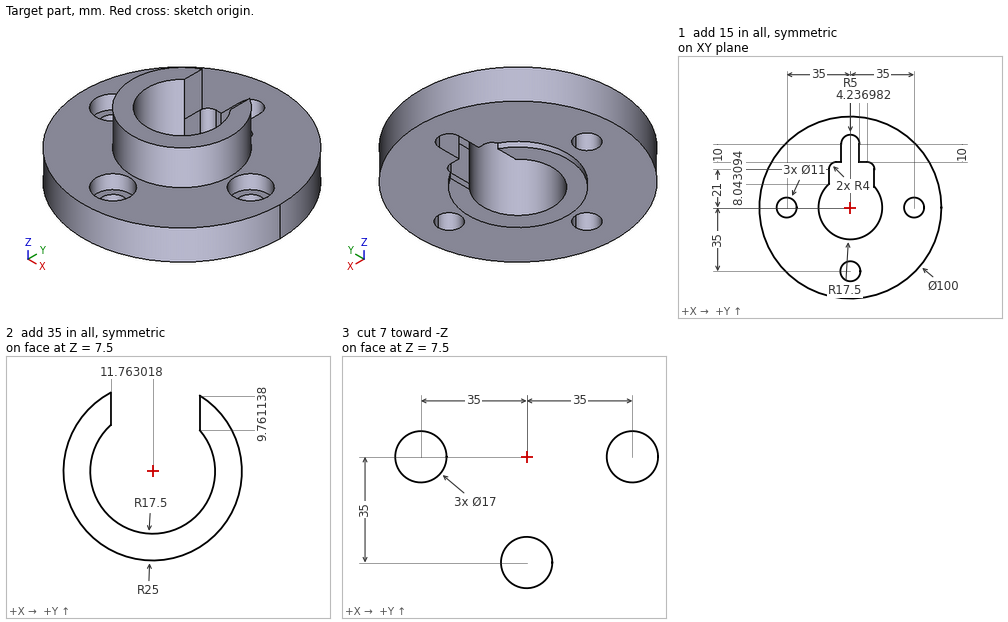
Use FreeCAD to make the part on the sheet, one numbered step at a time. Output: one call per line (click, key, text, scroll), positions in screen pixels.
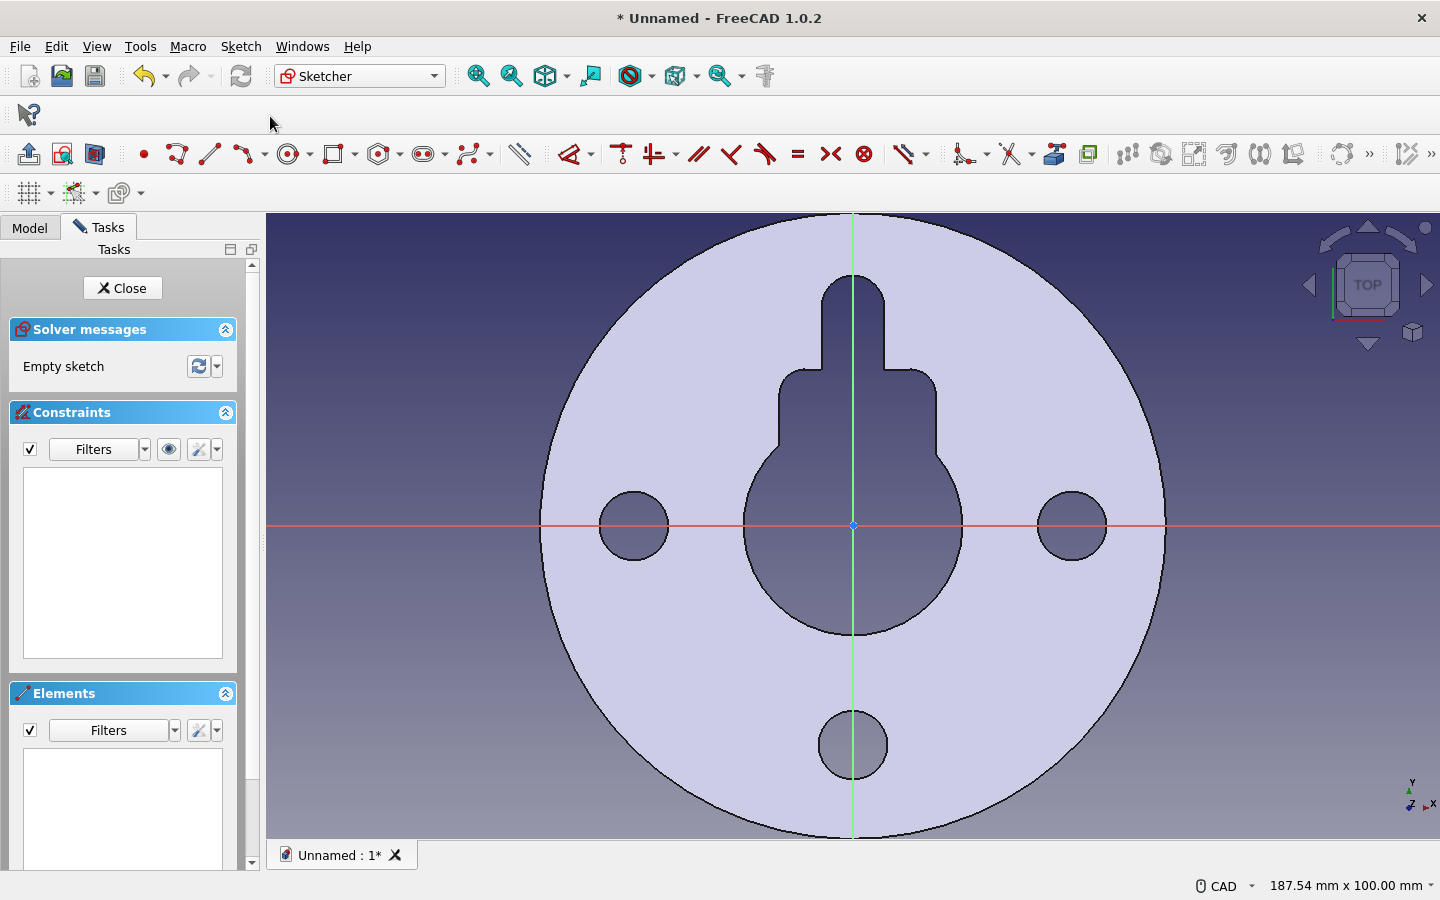
scroll(1006, 554, up, 2)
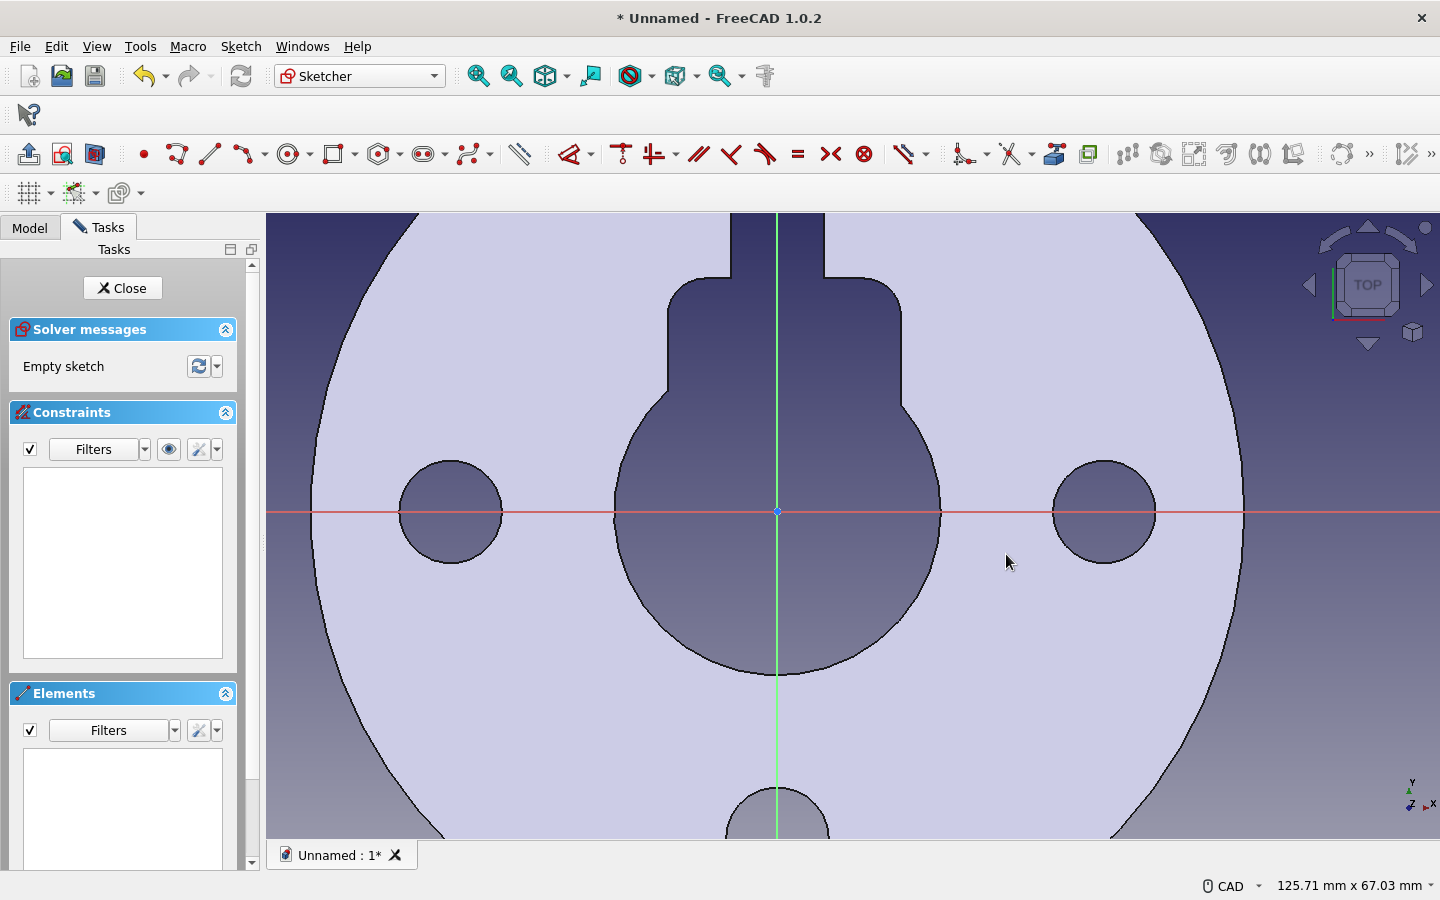
click(210, 154)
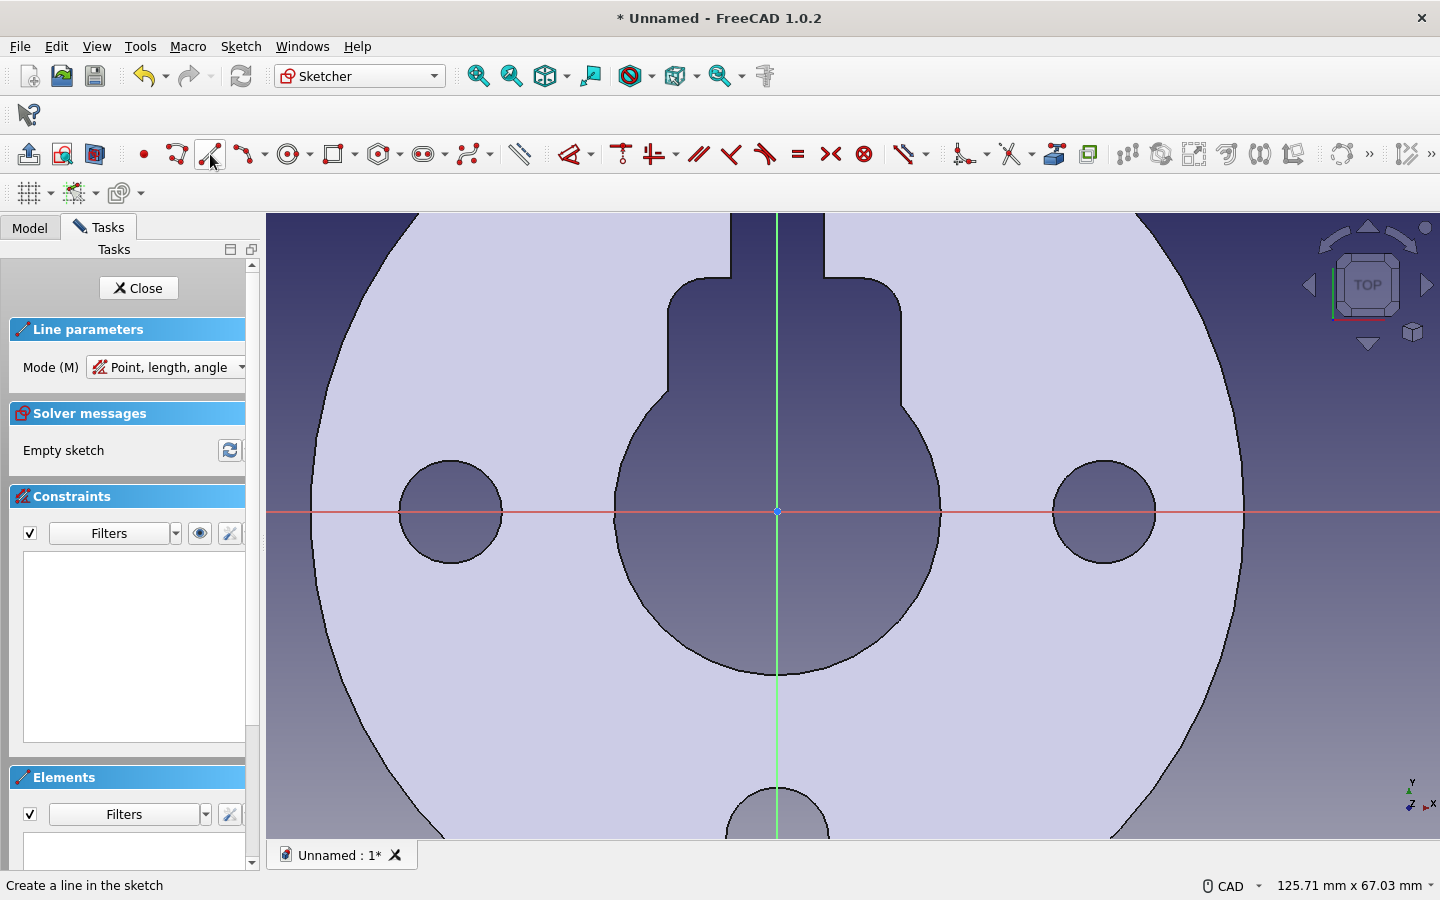
click(668, 391)
click(668, 306)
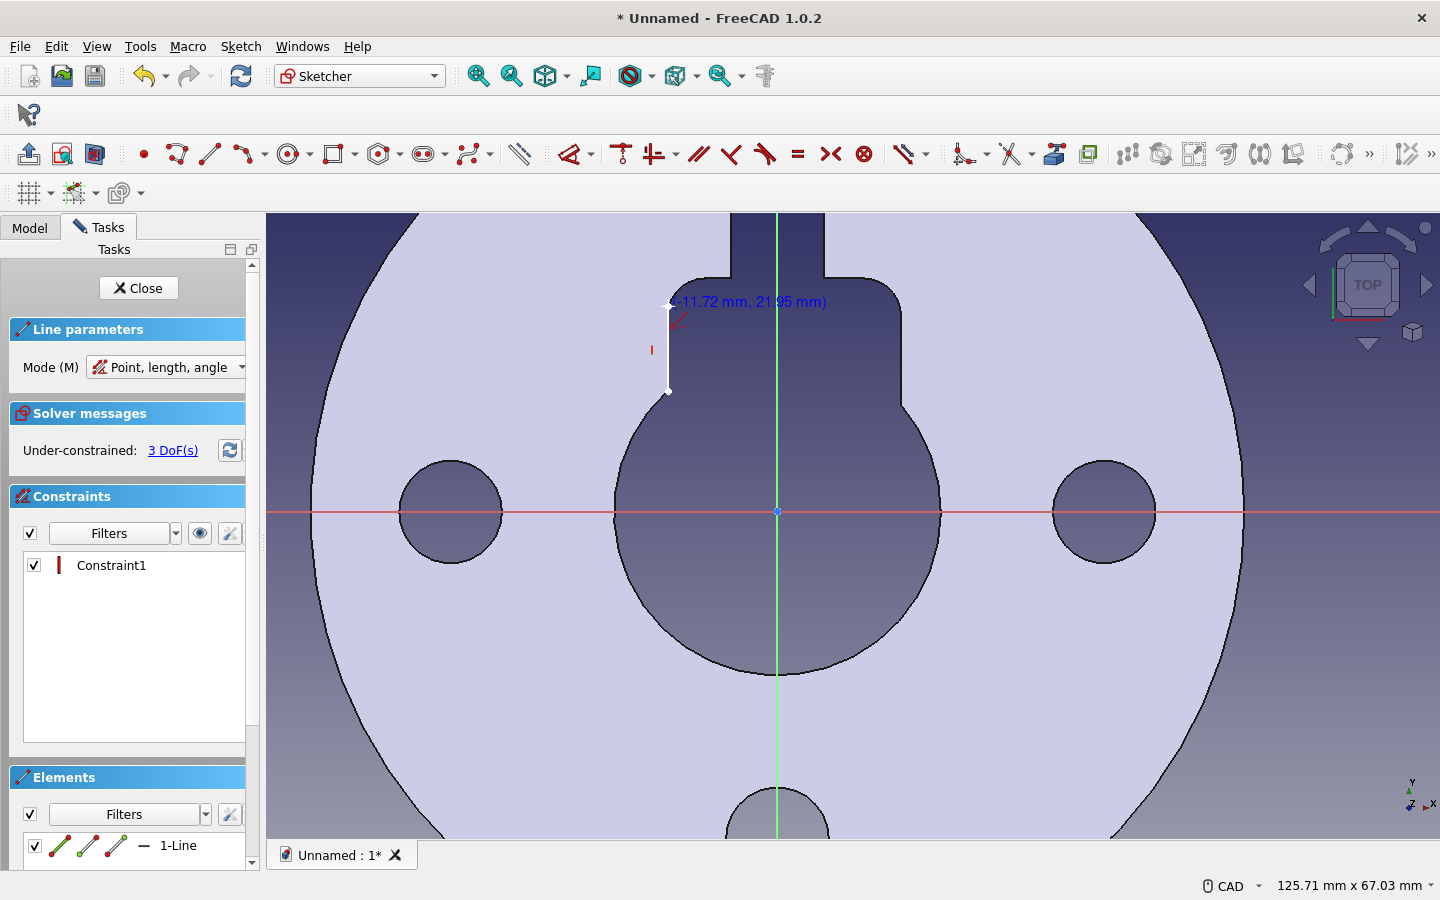
click(901, 314)
click(901, 405)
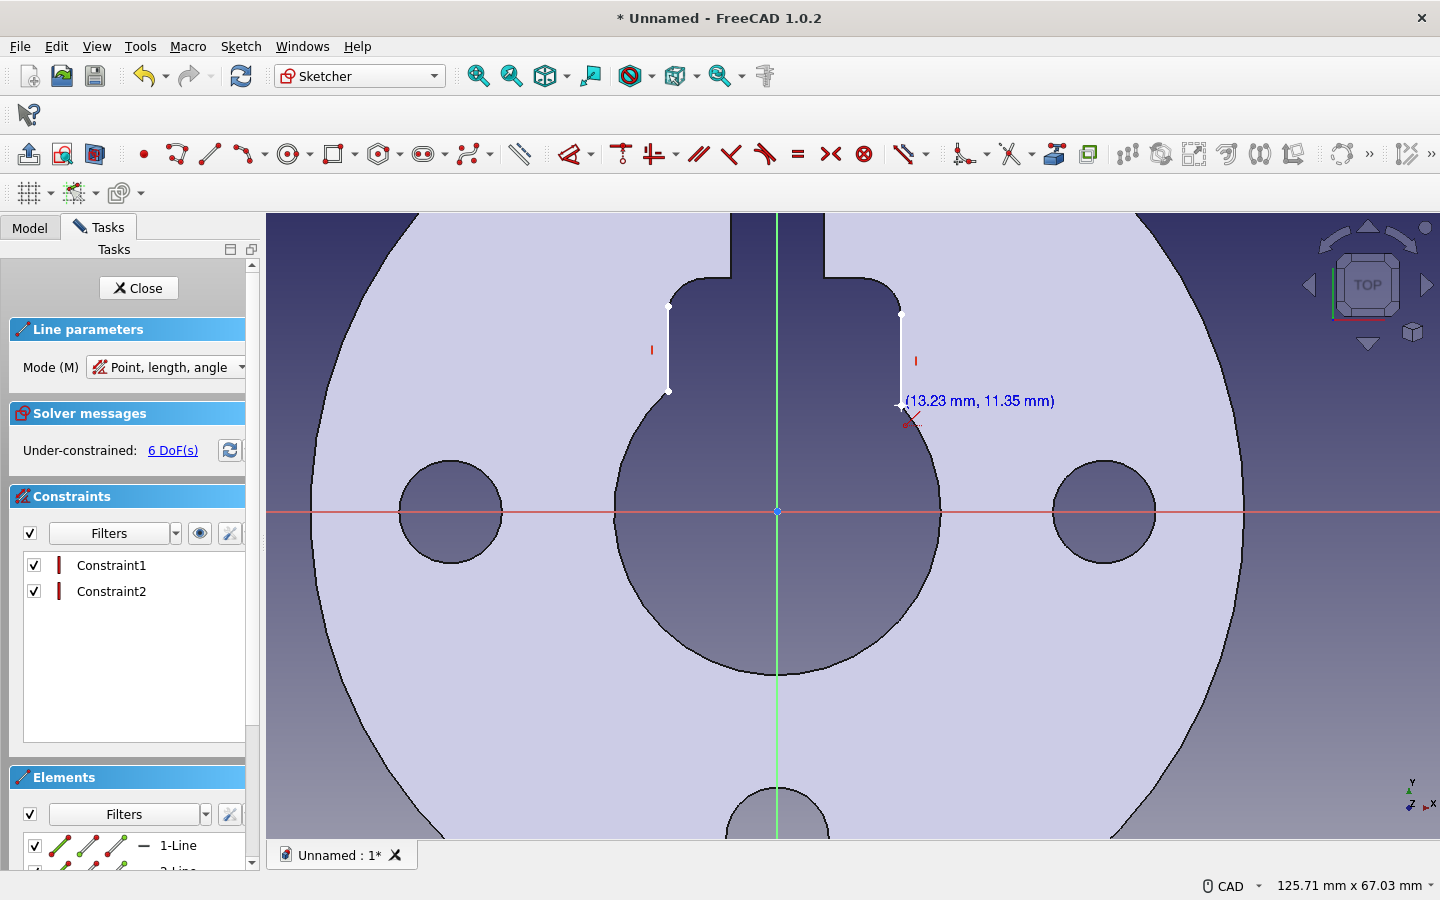
click(242, 154)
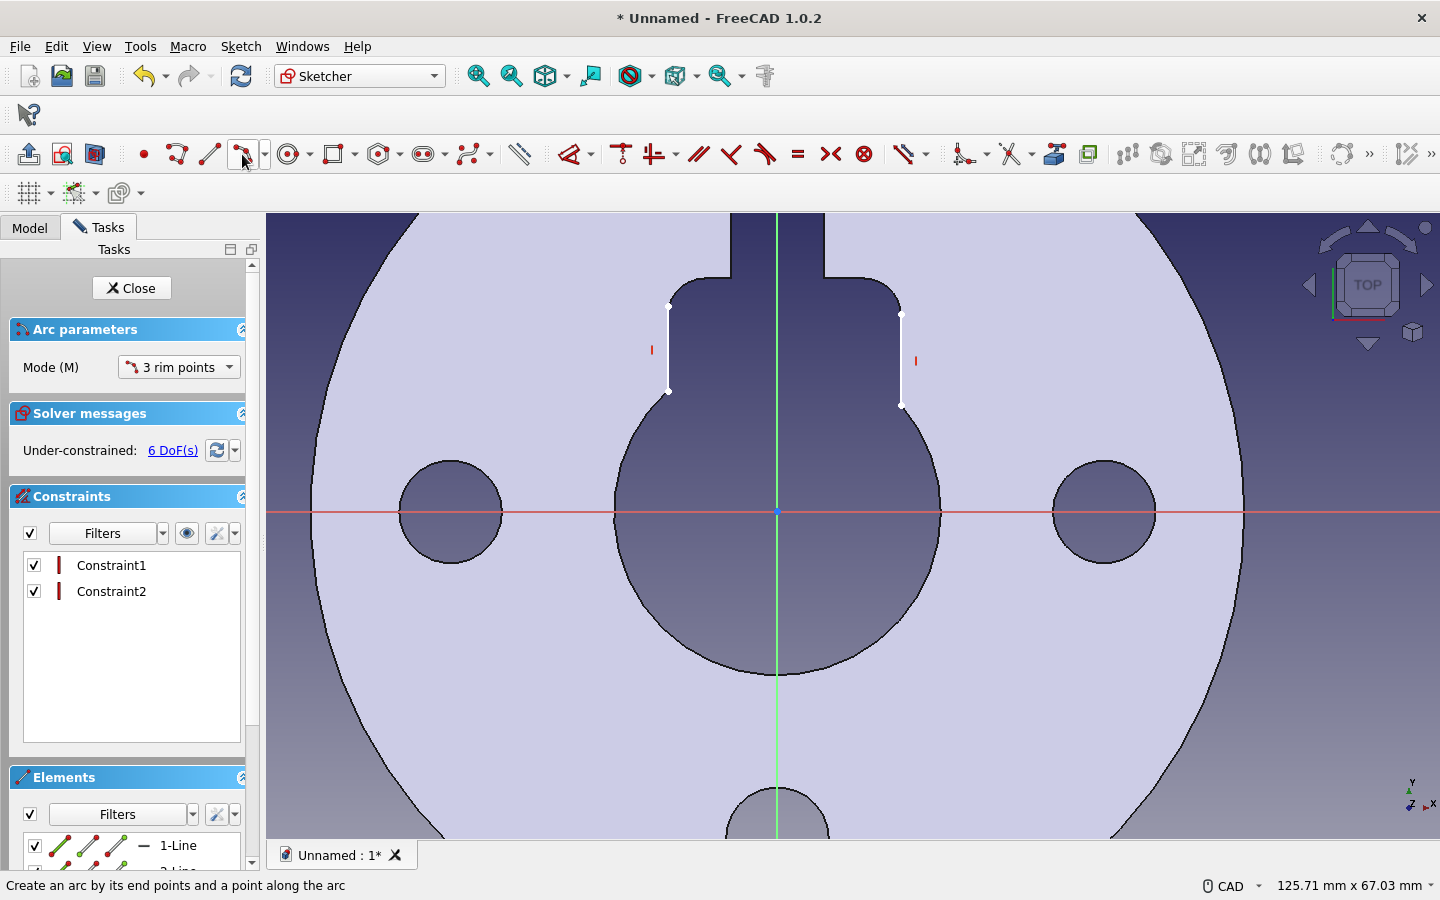
click(668, 307)
click(901, 315)
click(654, 710)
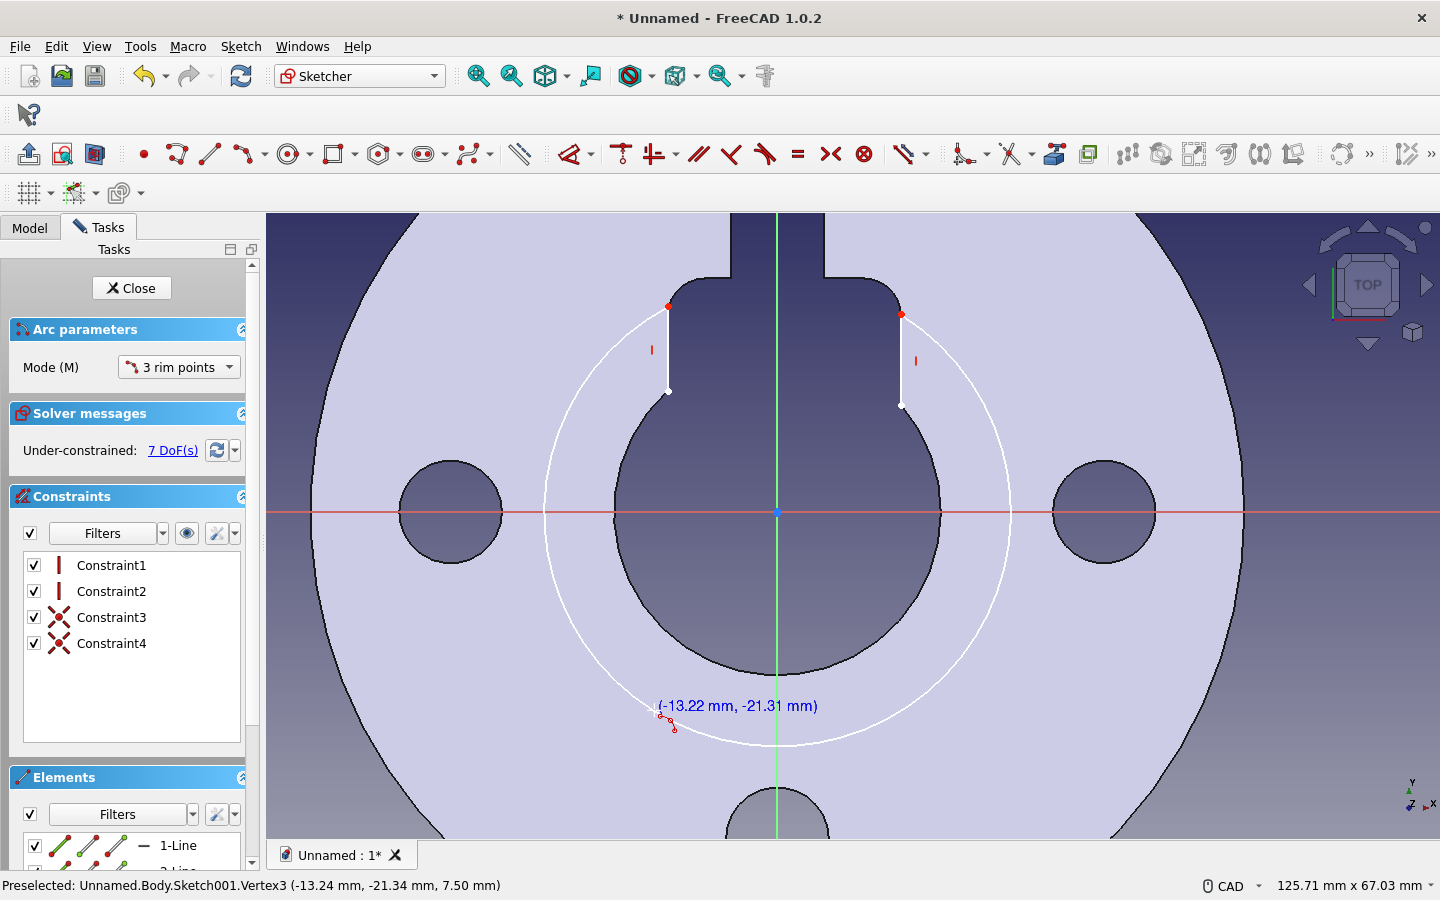
click(901, 406)
click(668, 392)
click(695, 653)
key(Escape)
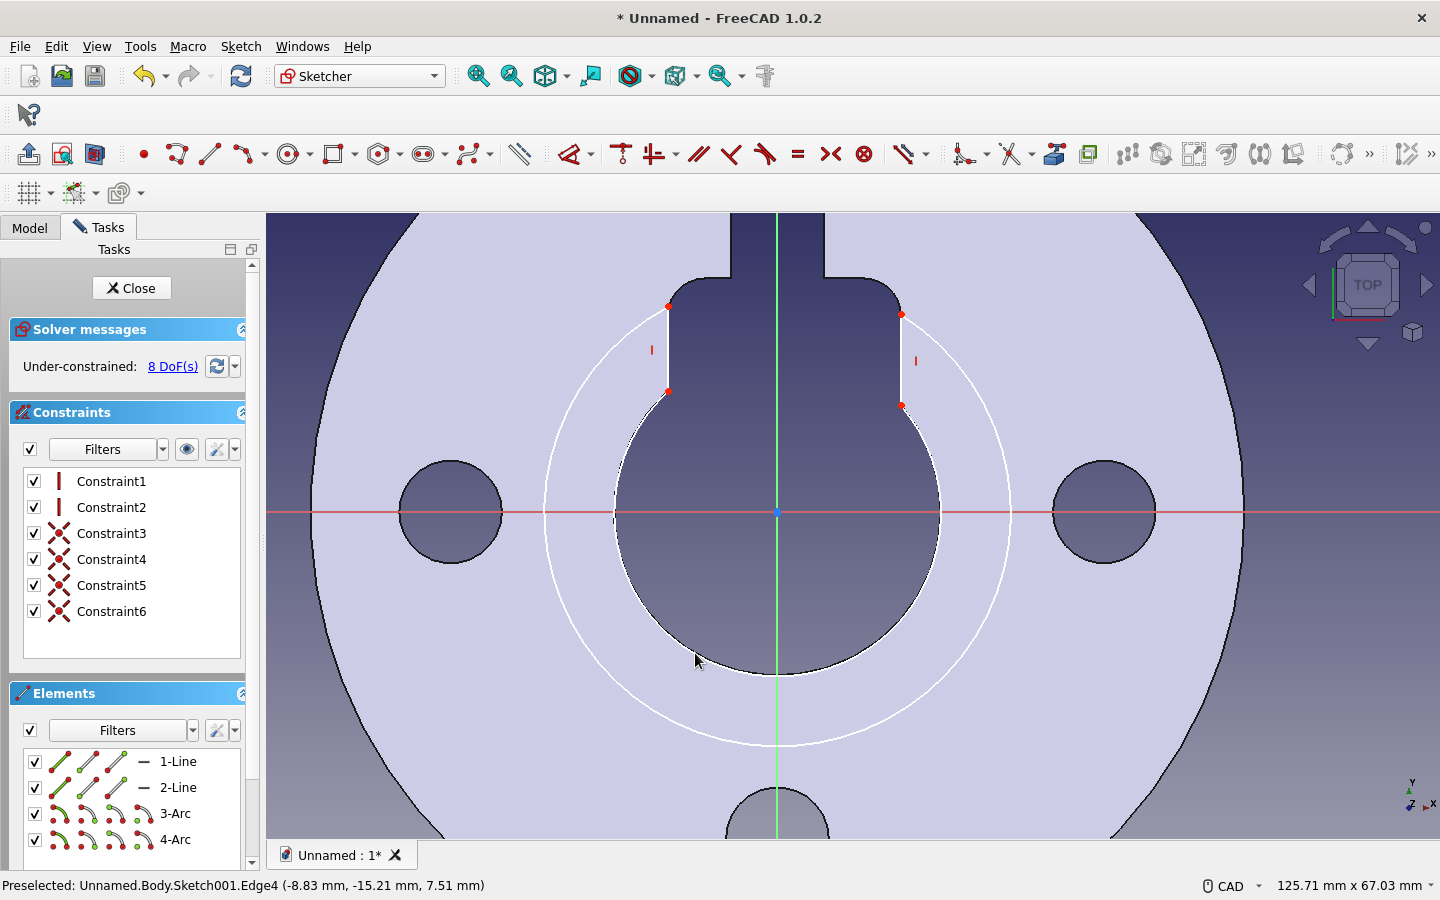
click(572, 623)